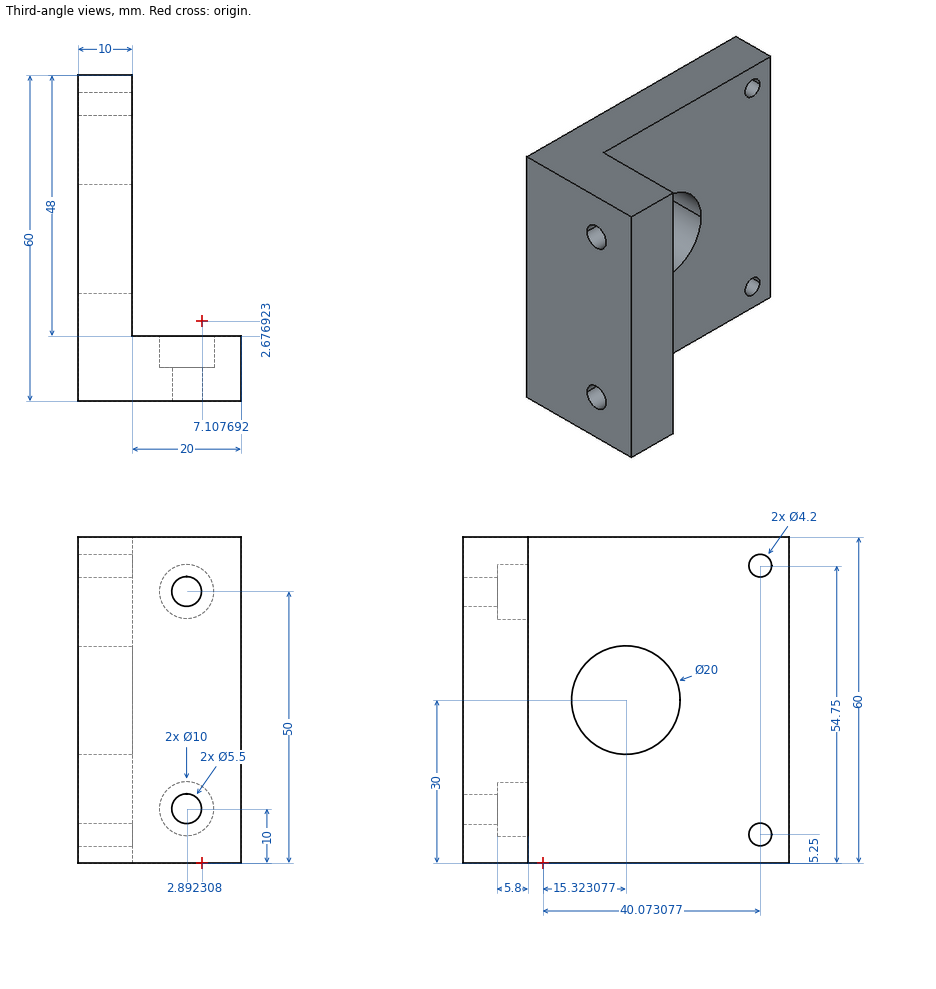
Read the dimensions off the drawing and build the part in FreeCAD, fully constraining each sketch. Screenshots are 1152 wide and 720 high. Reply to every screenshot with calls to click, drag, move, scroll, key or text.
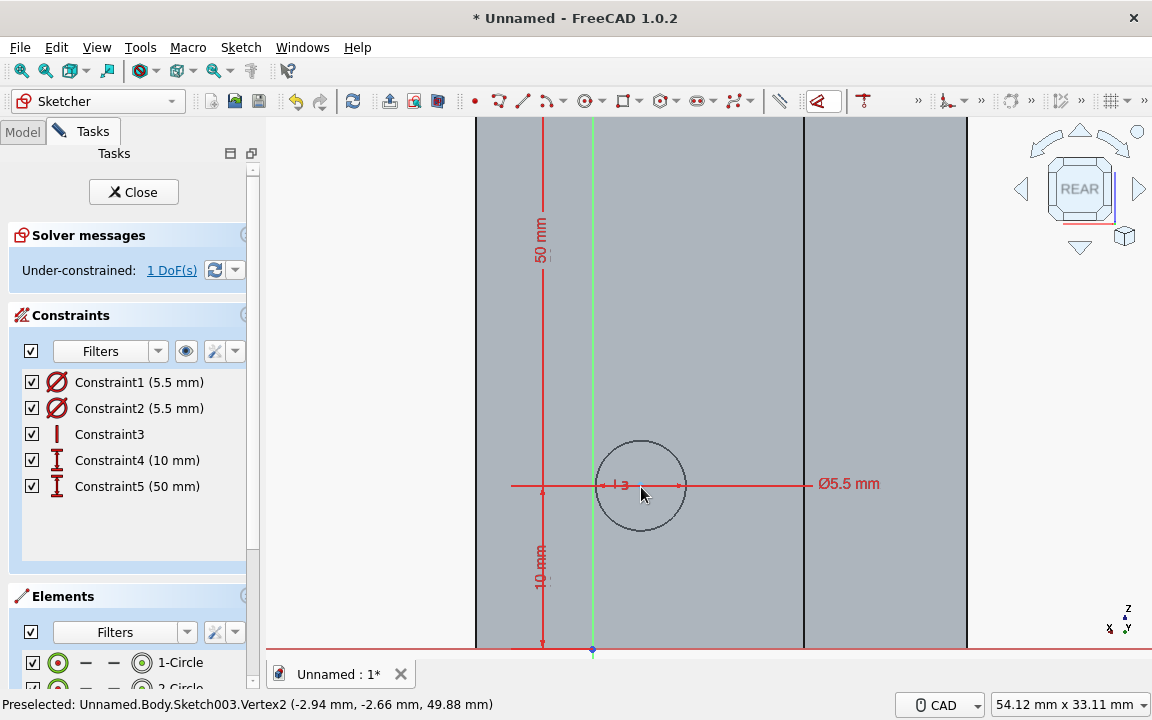
click(641, 486)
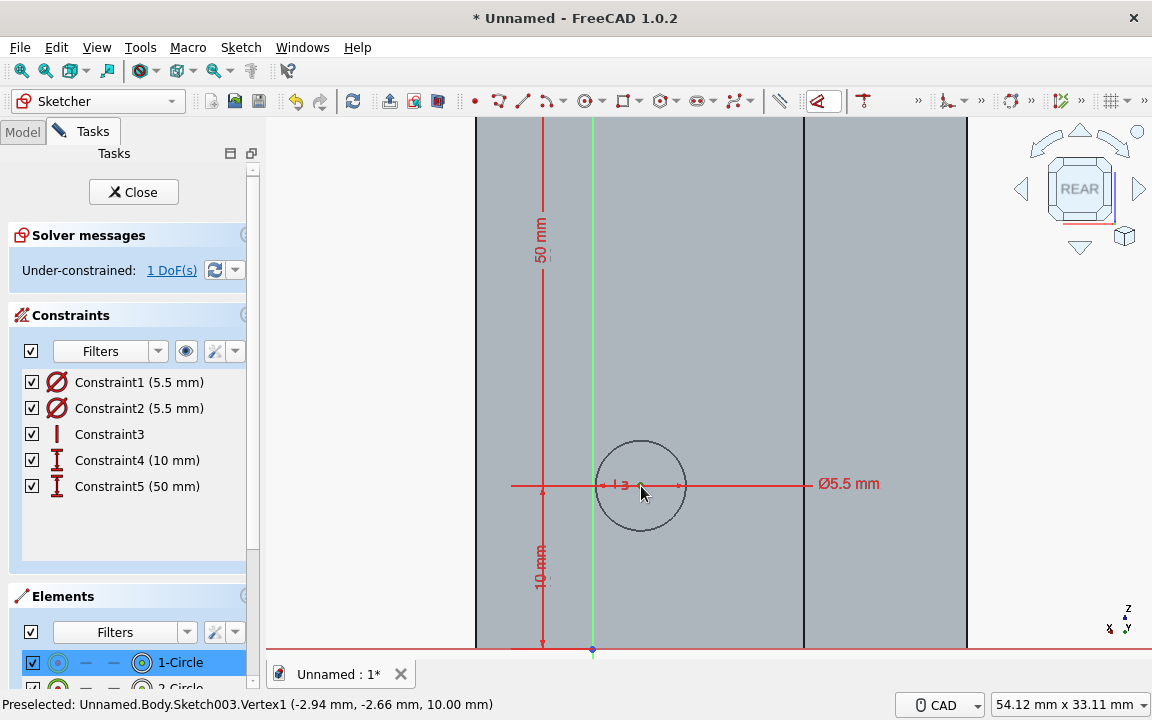
click(836, 102)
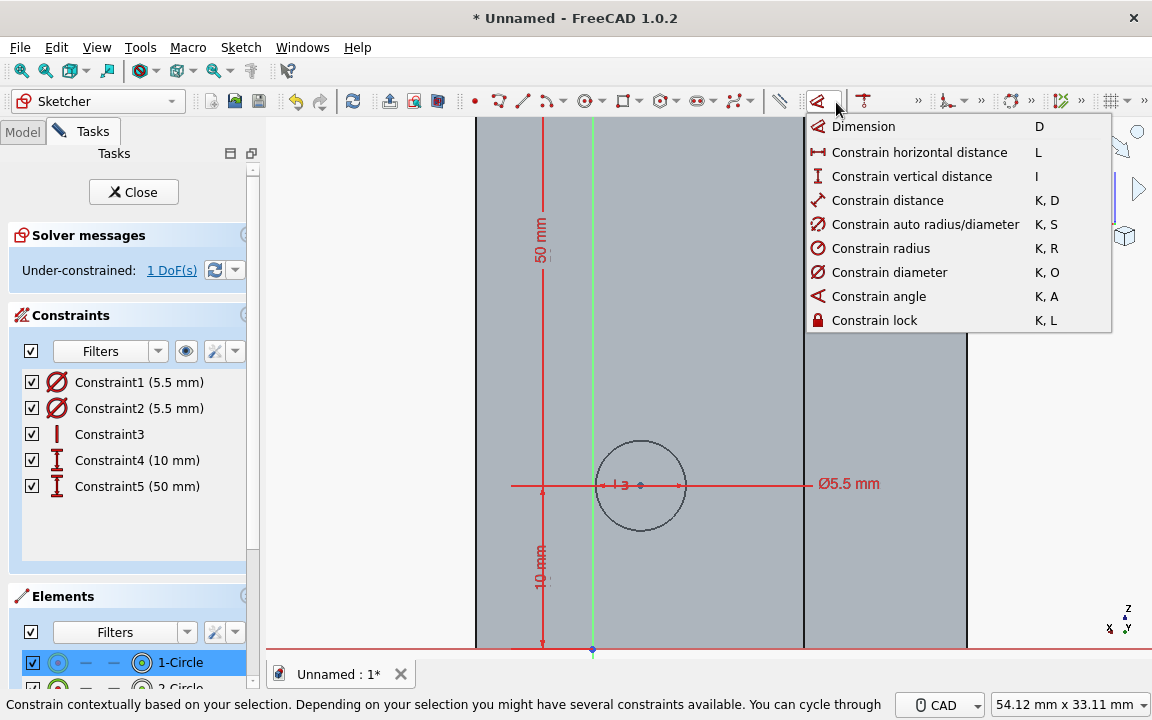
click(959, 152)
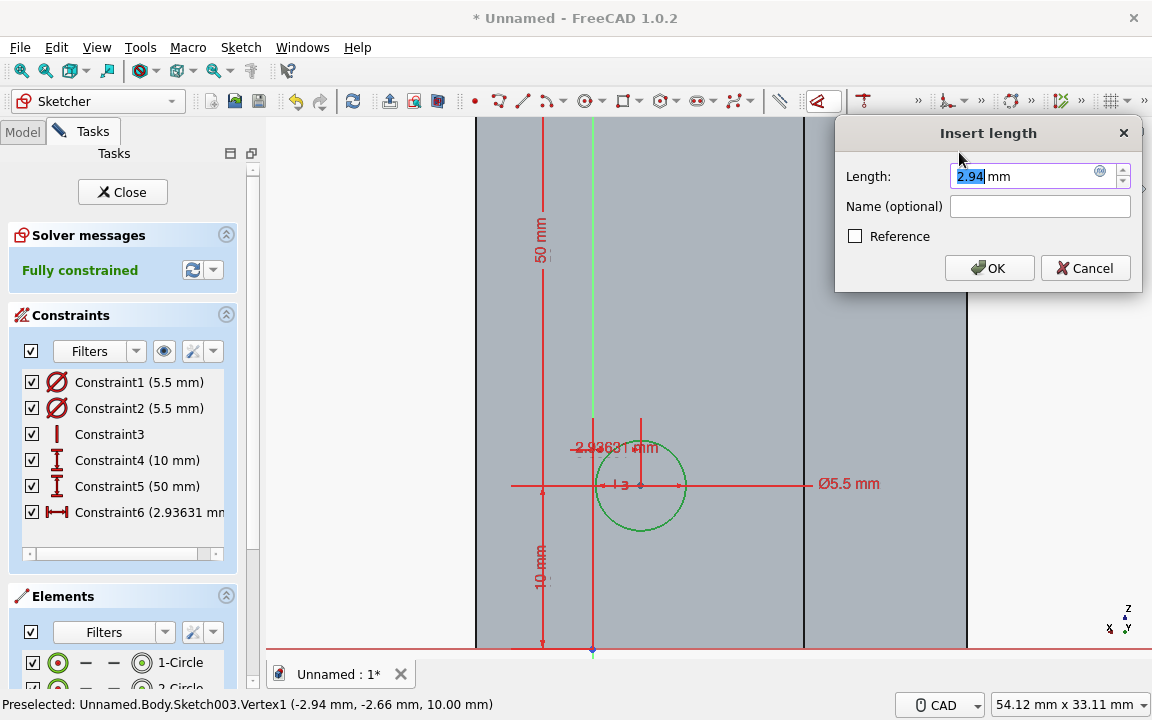
text(2.892308)
key(Return)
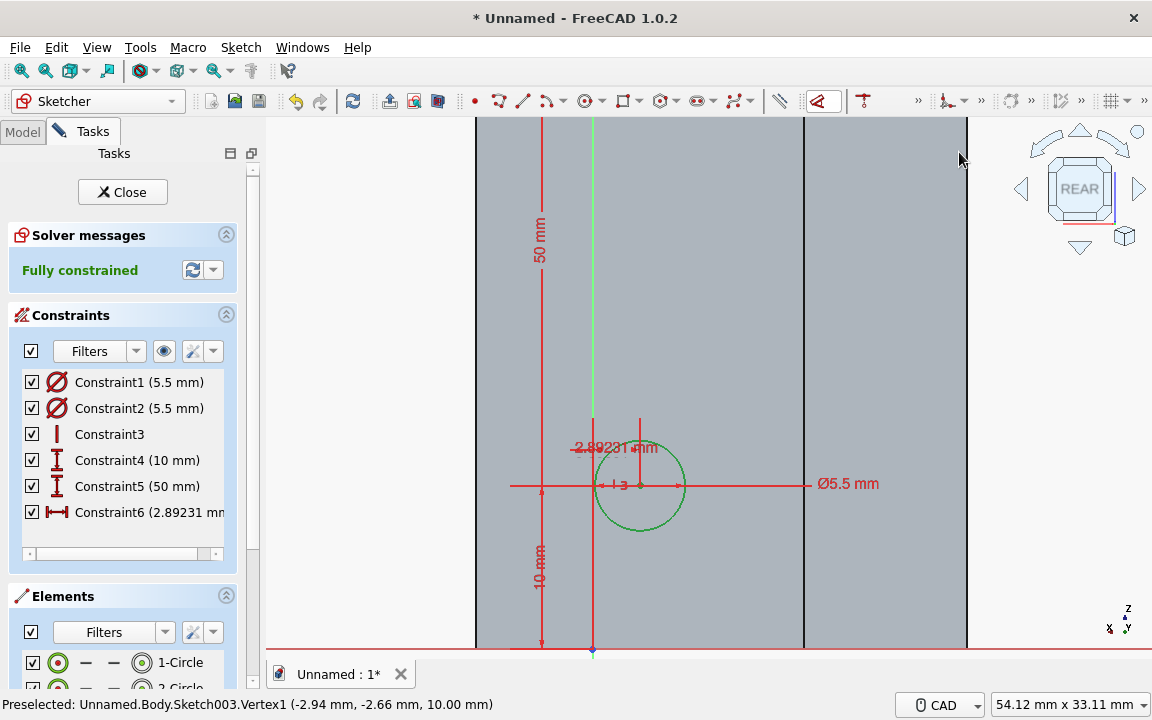
click(123, 192)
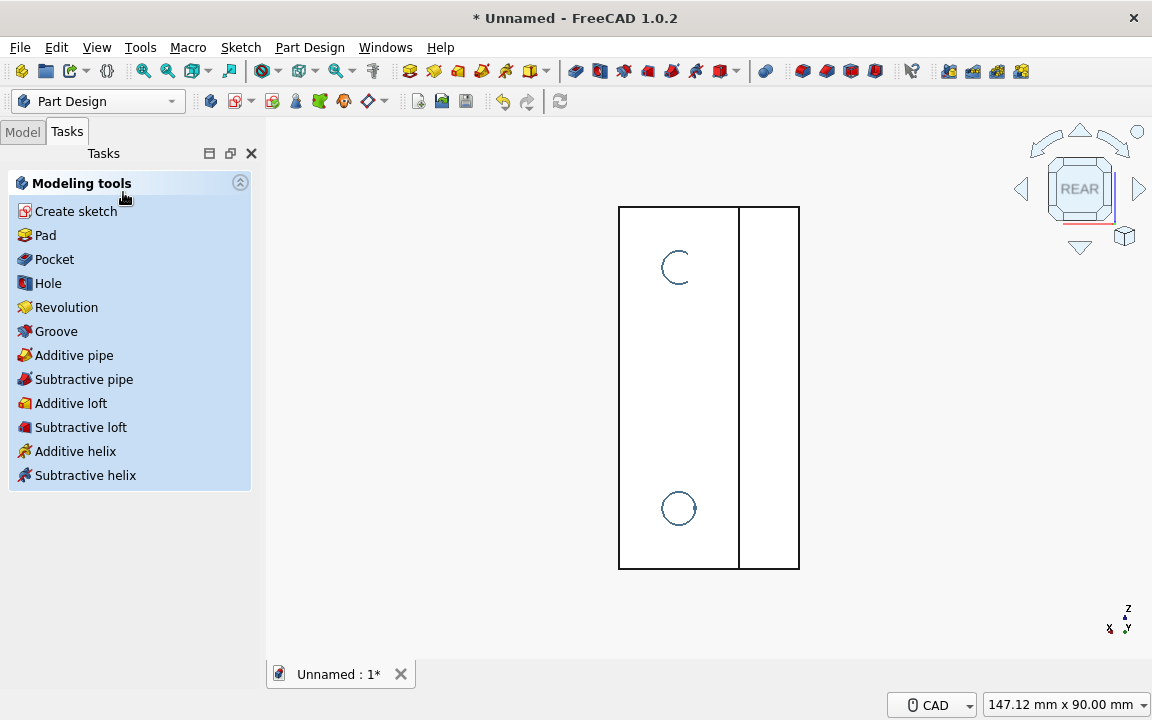
click(576, 72)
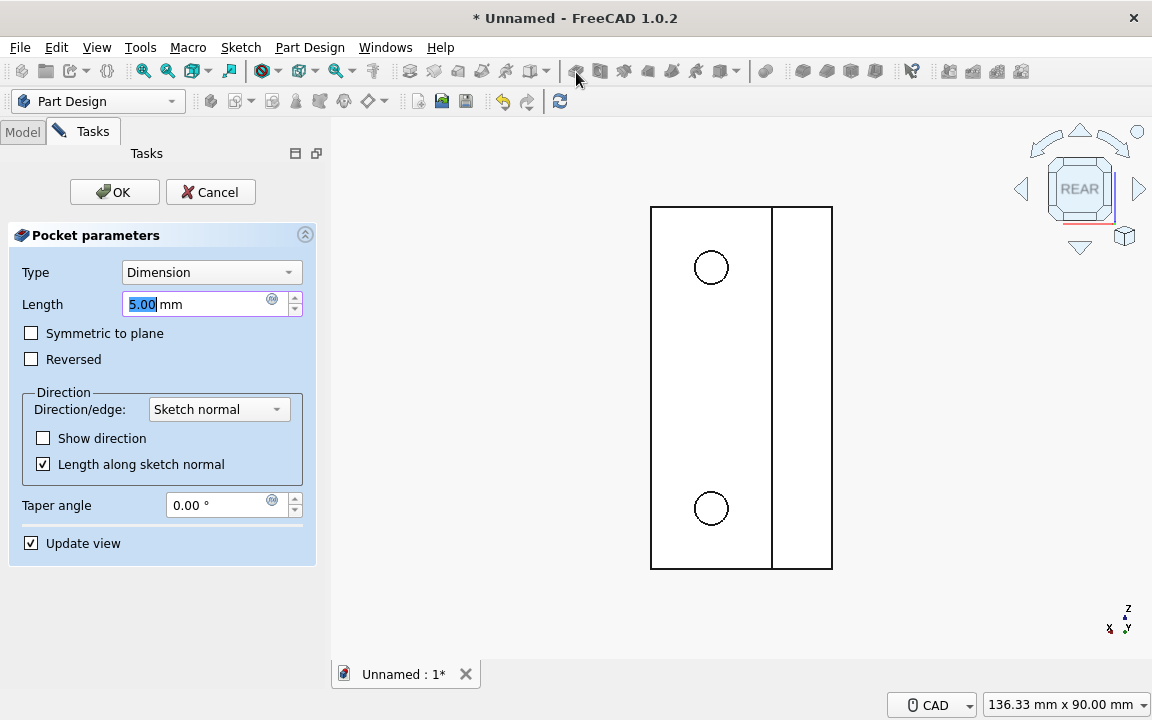
click(212, 272)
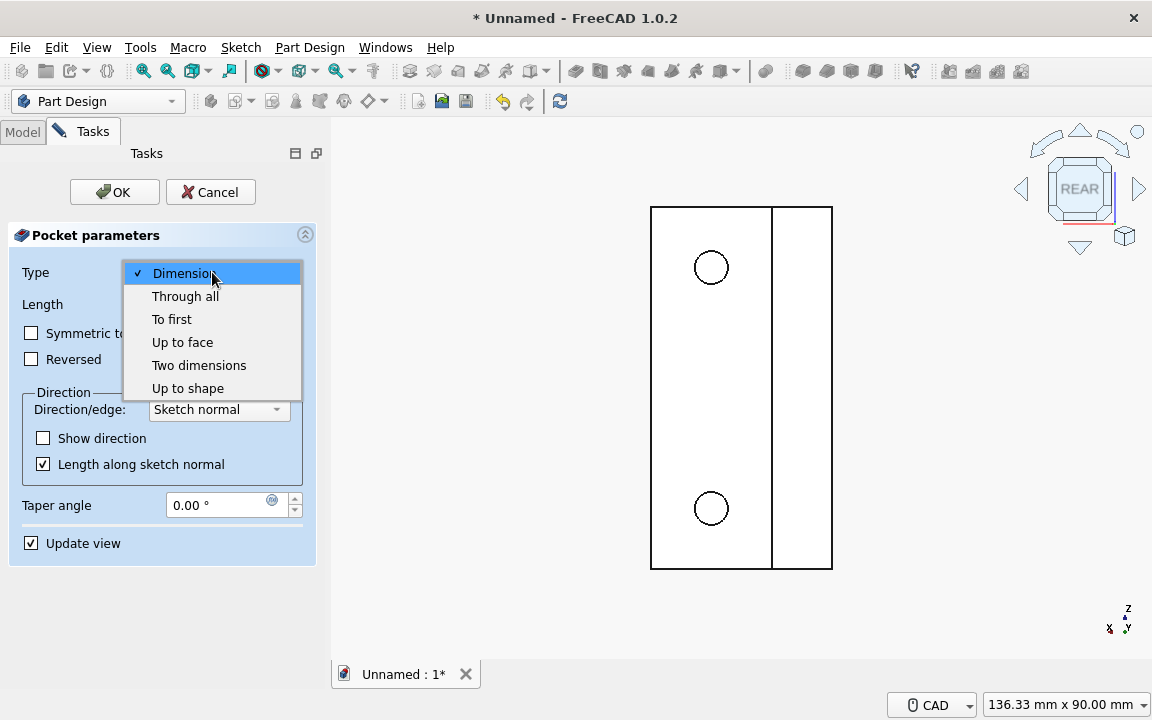
click(212, 296)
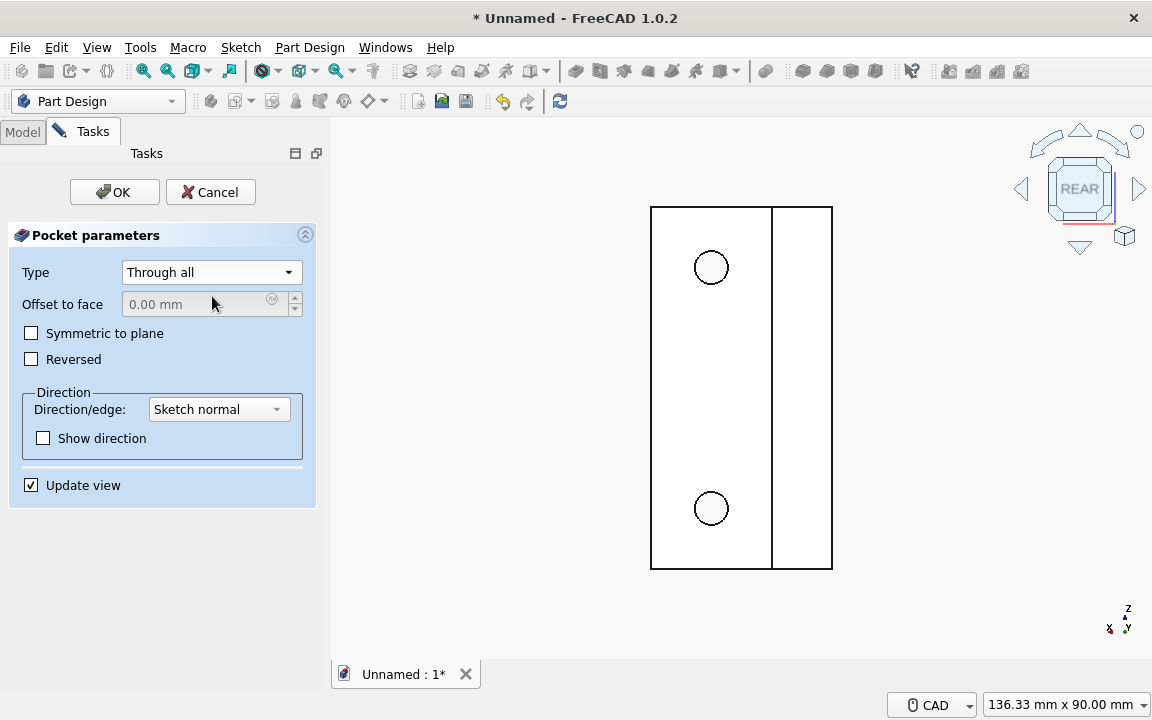
click(115, 192)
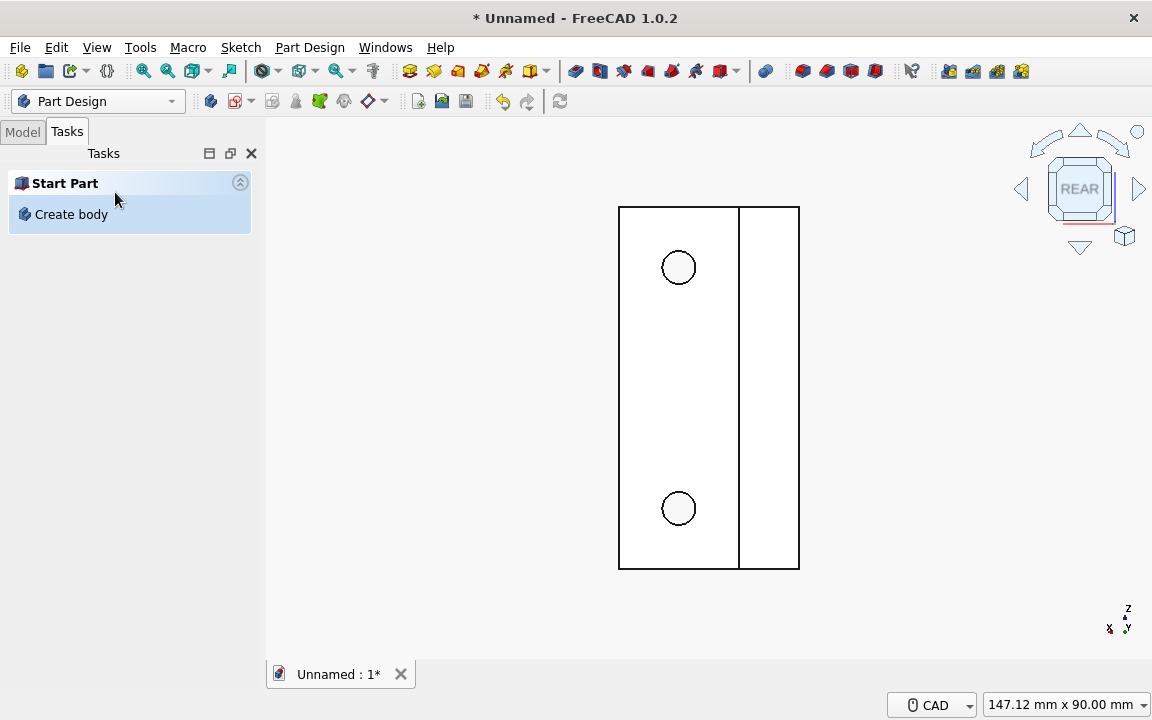
click(679, 387)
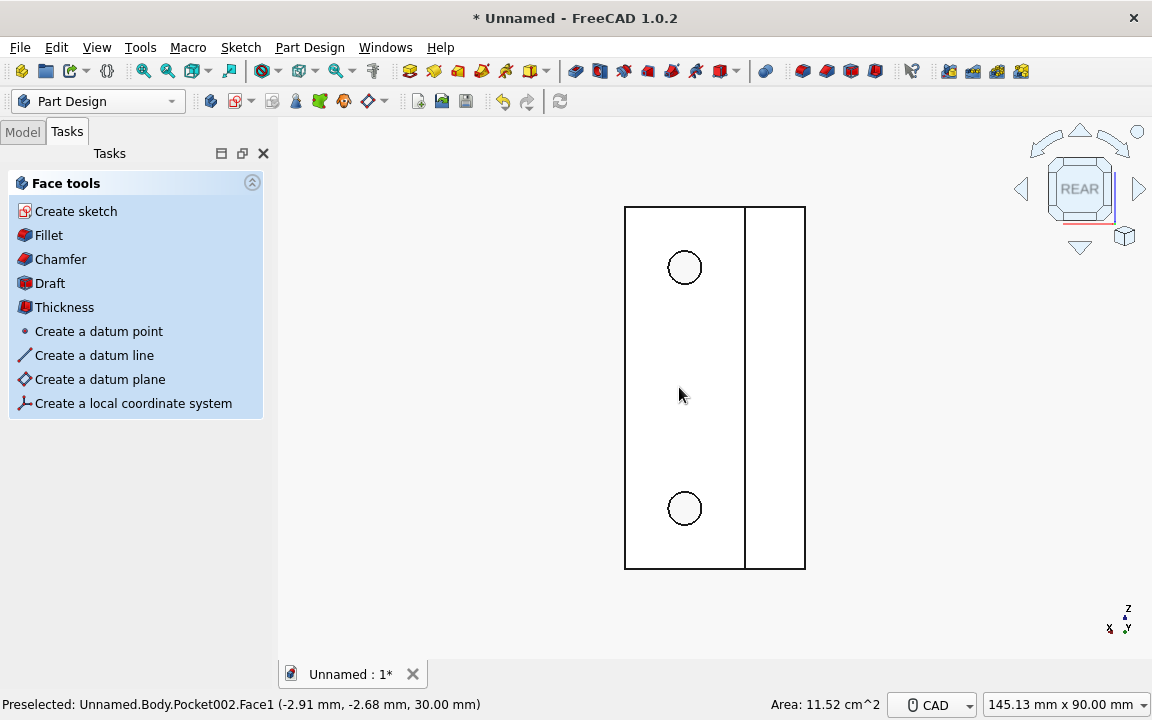
click(236, 102)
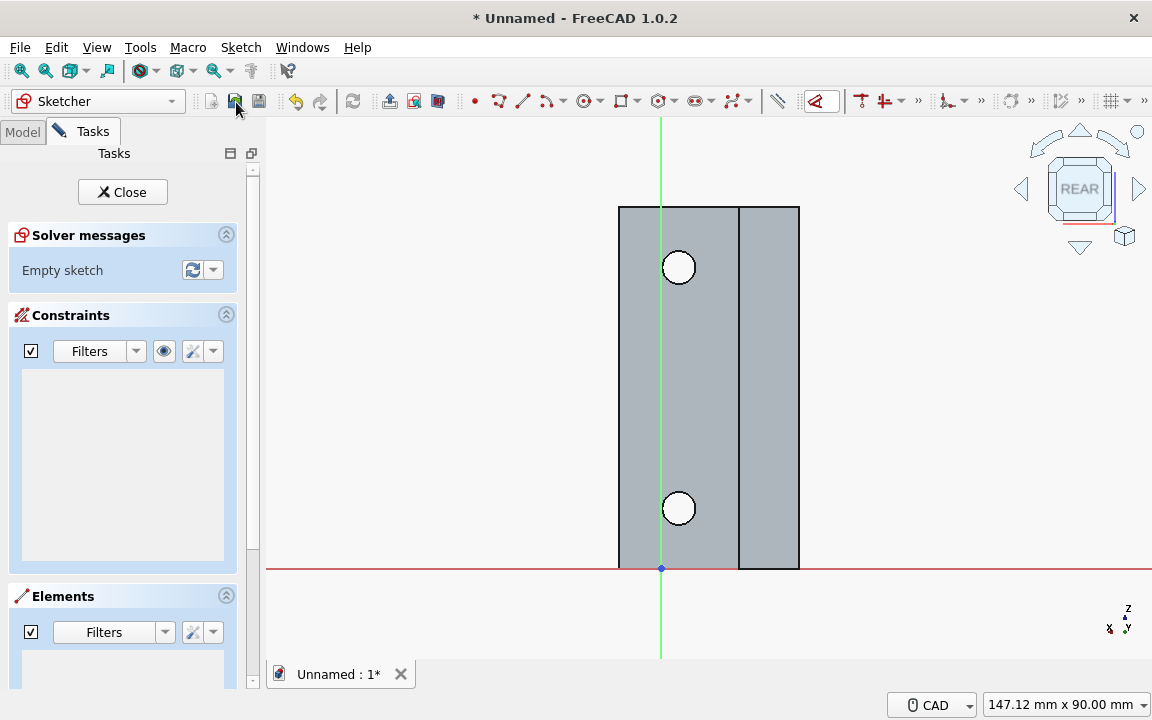
click(584, 102)